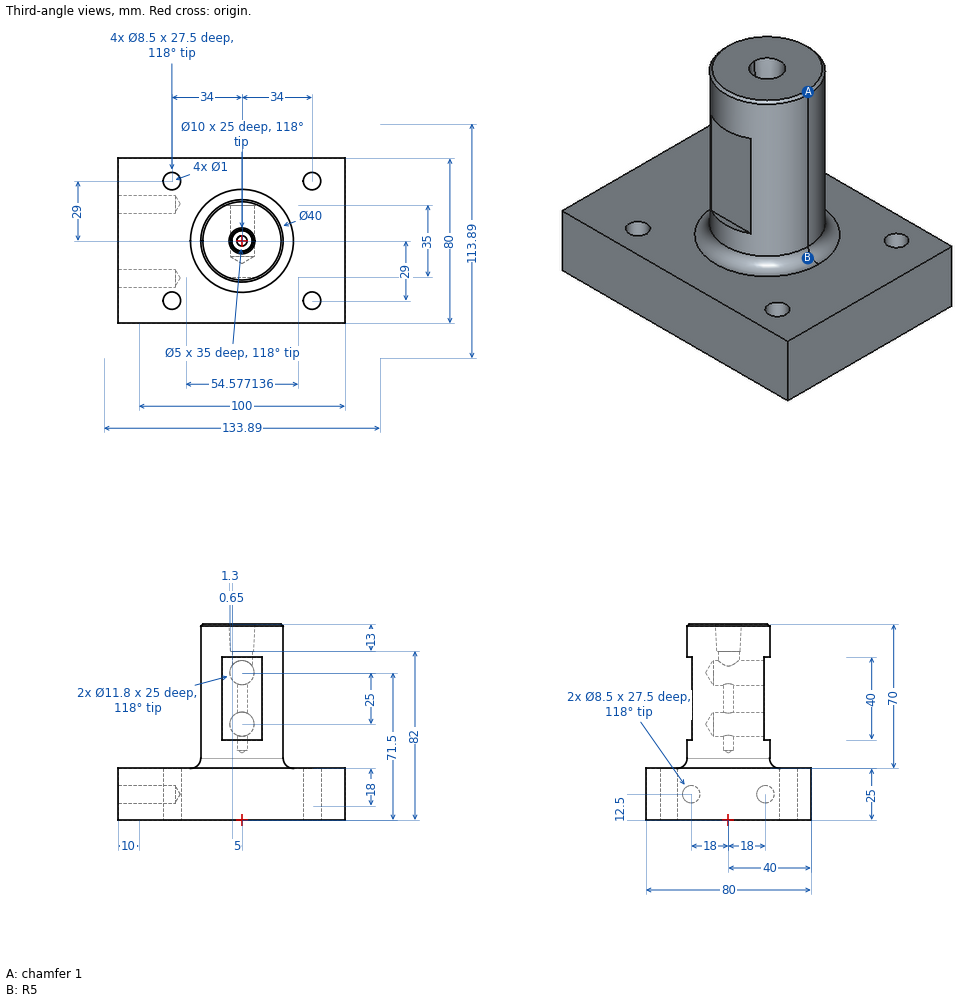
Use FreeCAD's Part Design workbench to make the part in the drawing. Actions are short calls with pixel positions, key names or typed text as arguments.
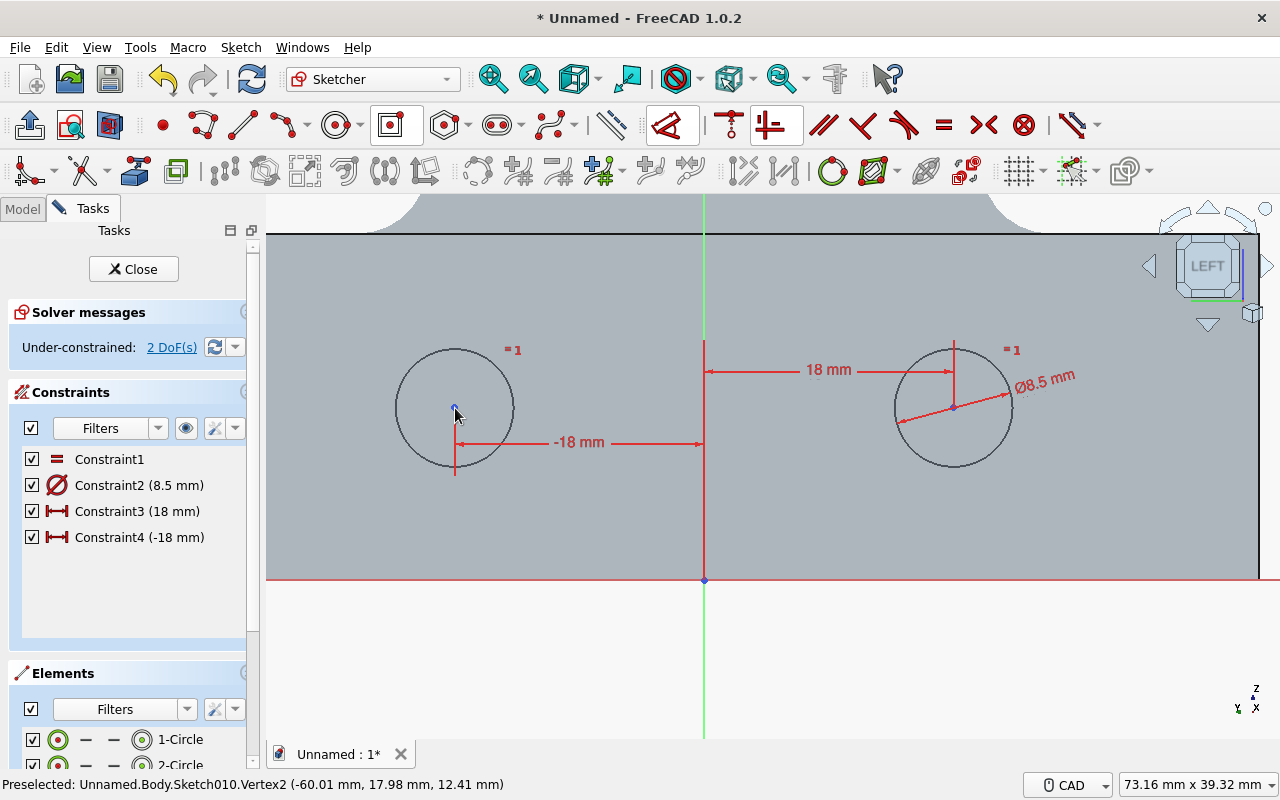
click(954, 408)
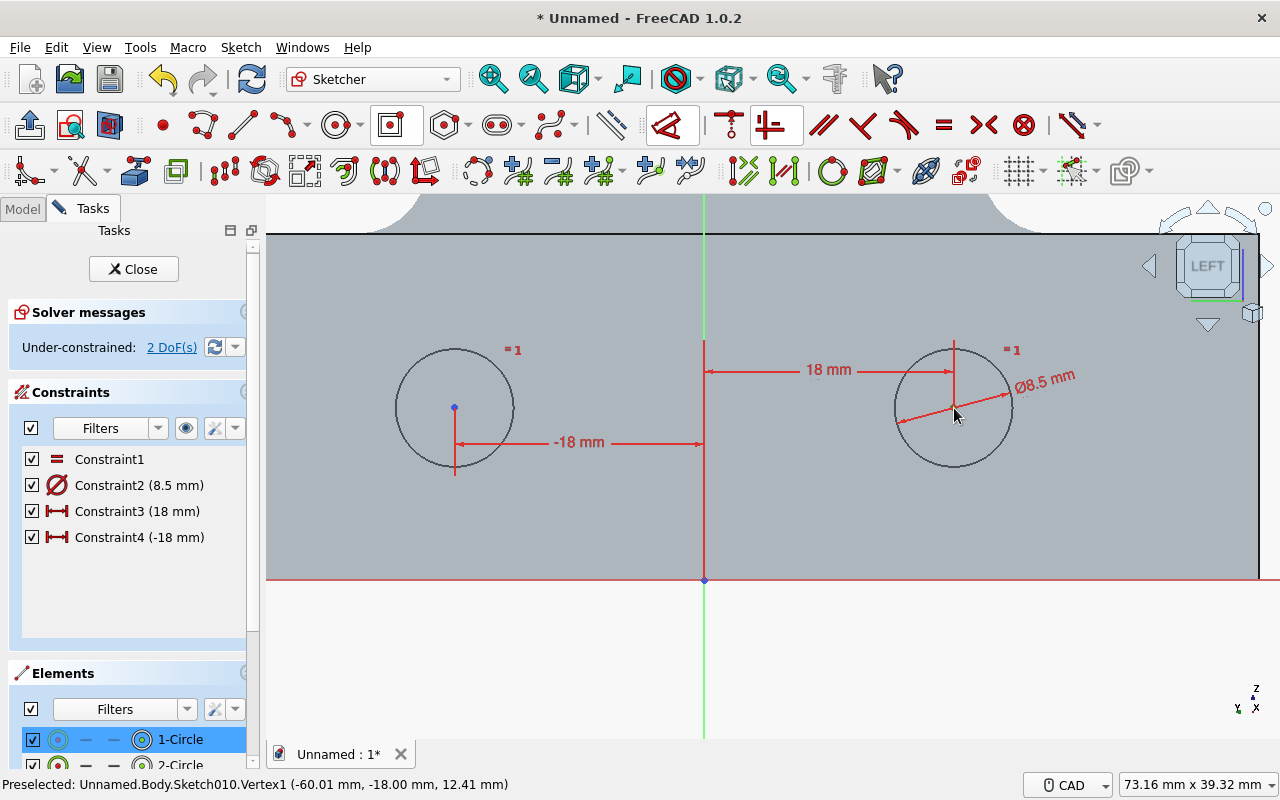
click(694, 126)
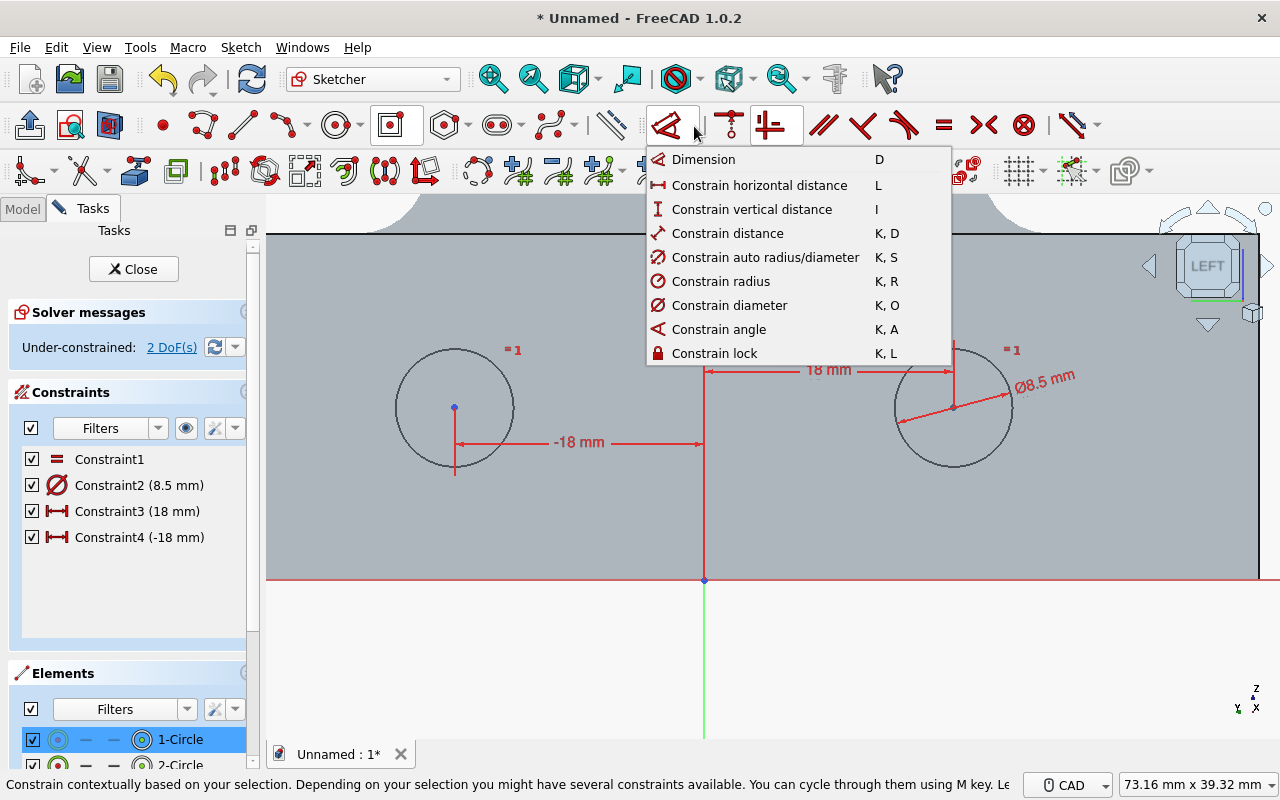
click(799, 209)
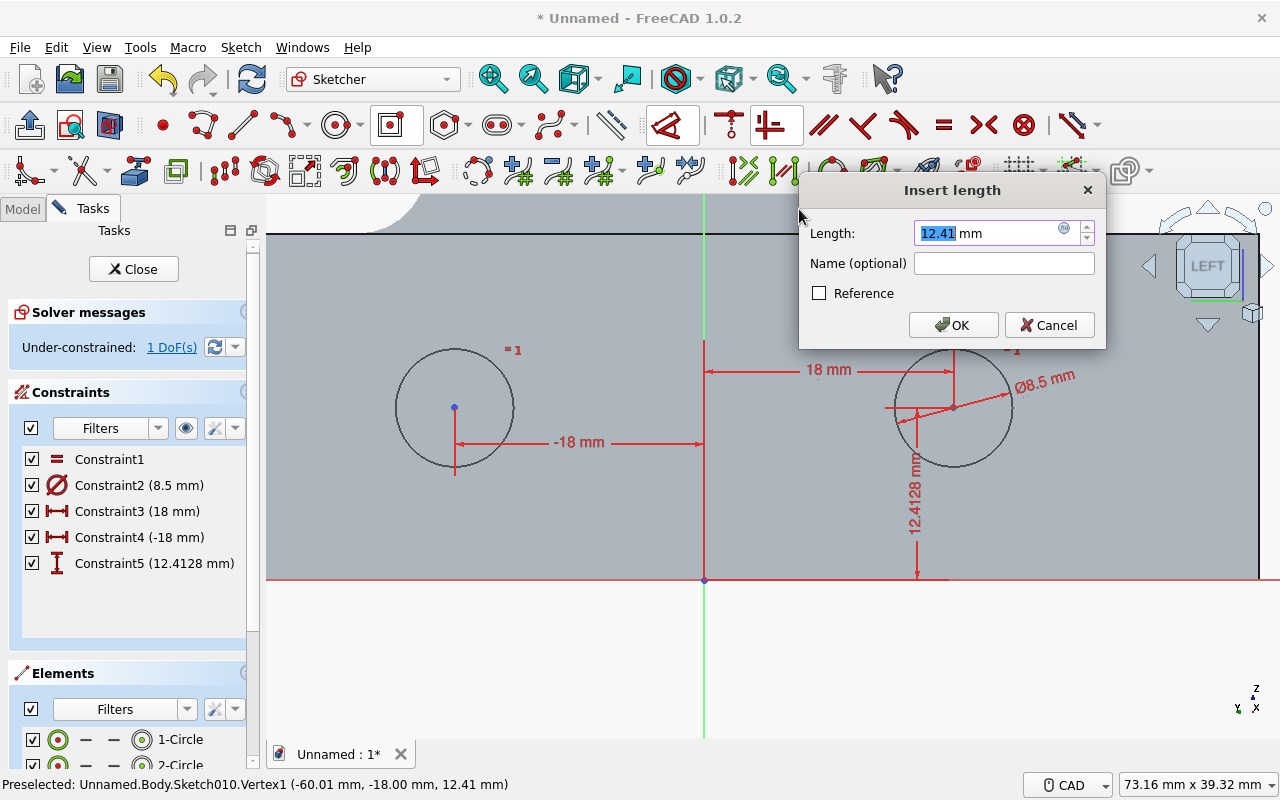
text(12.5)
key(Return)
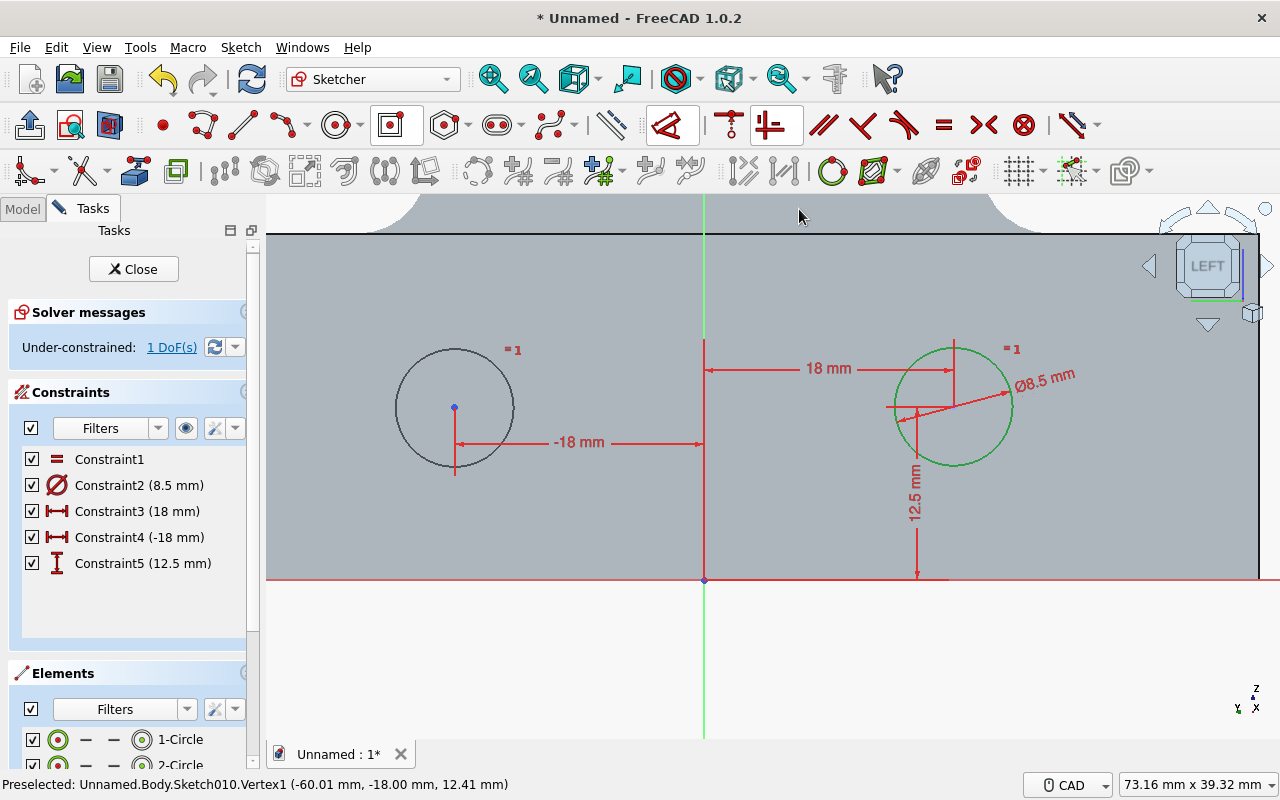
click(455, 408)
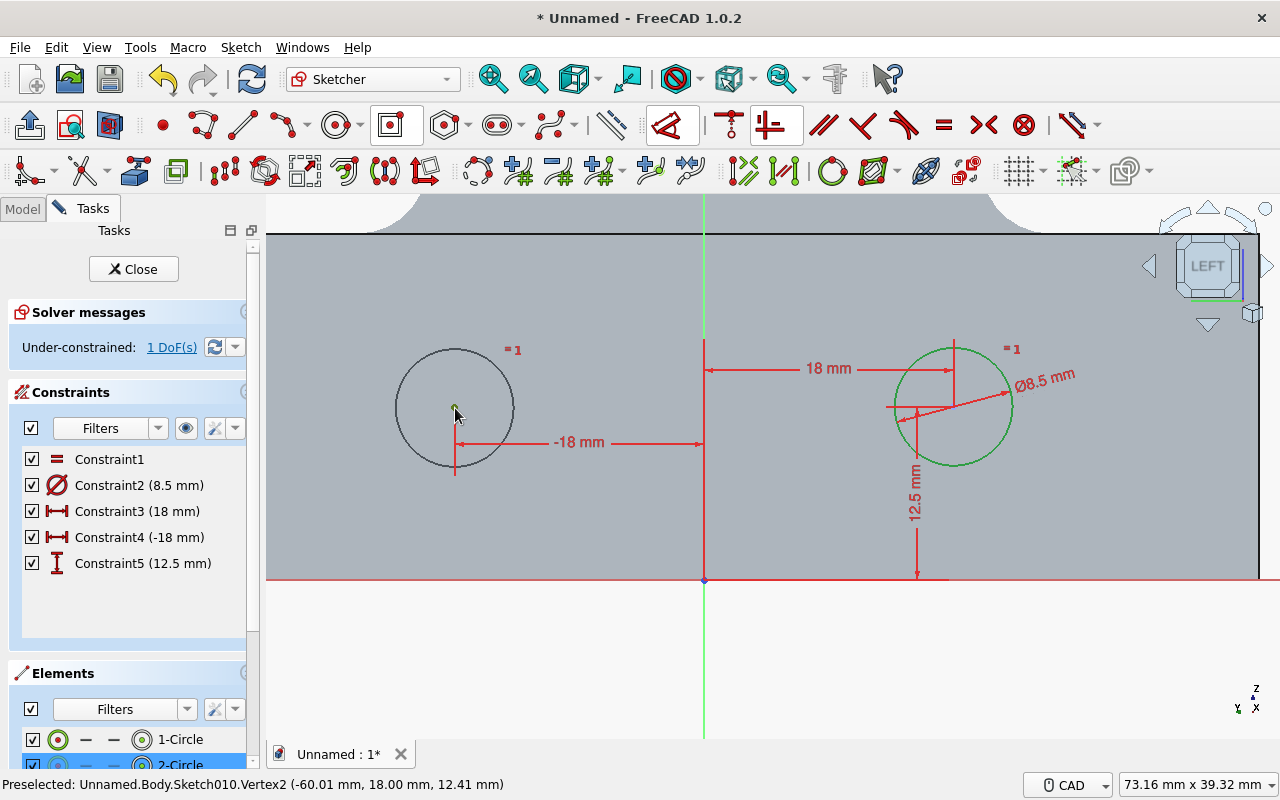
click(694, 126)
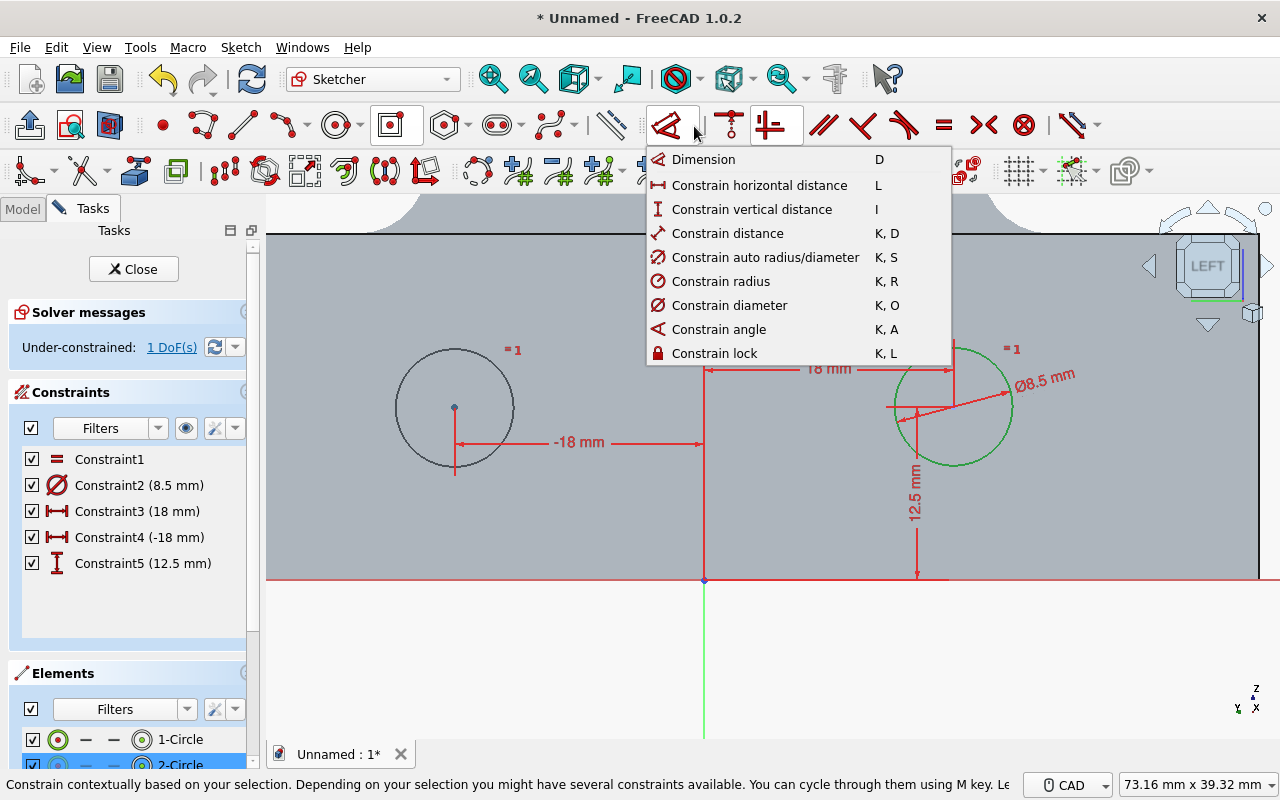
click(799, 209)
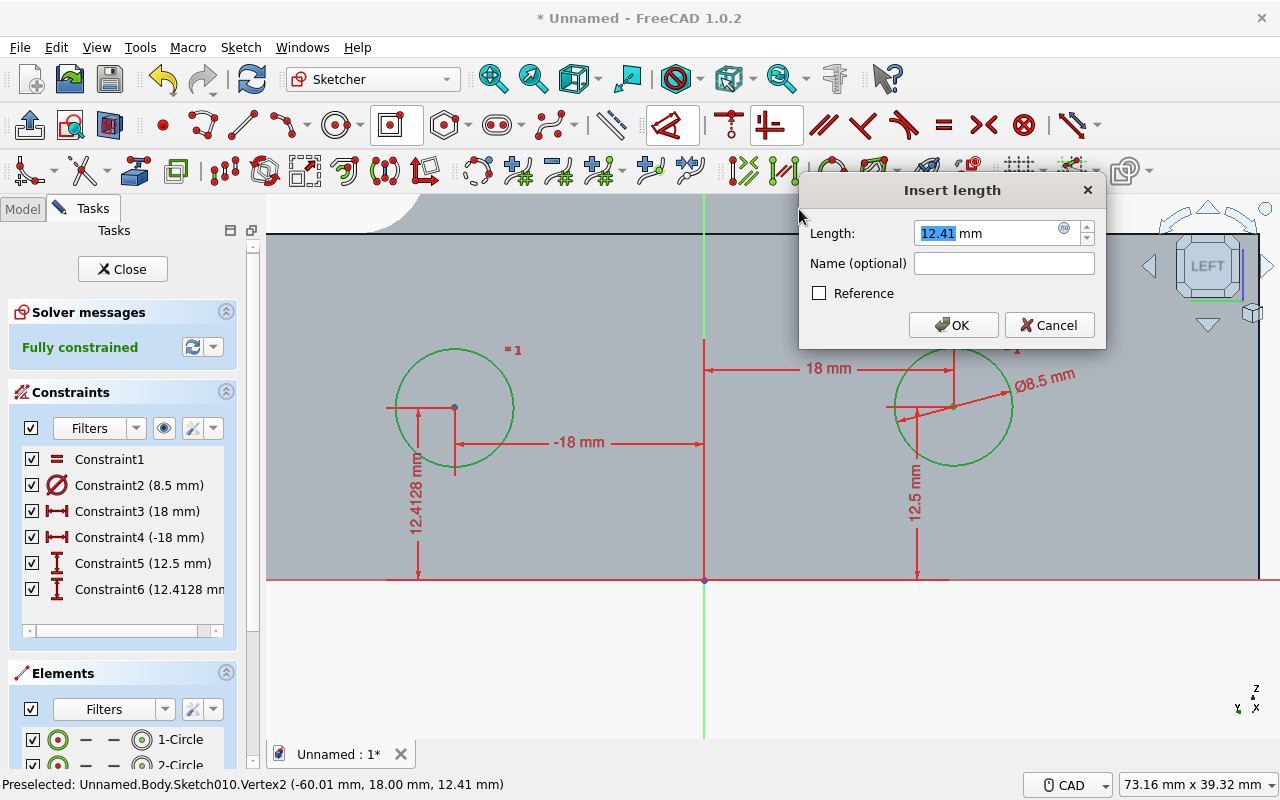
text(12.5)
key(Return)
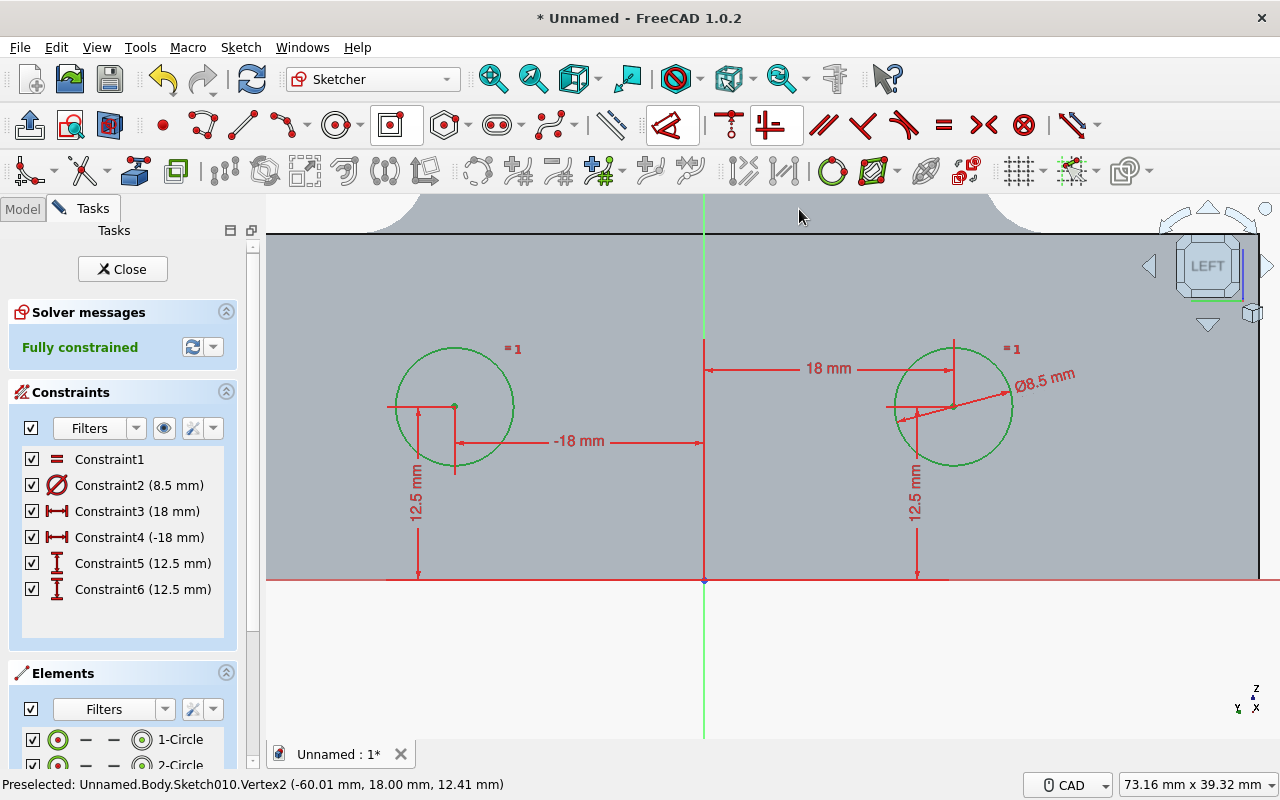
click(123, 269)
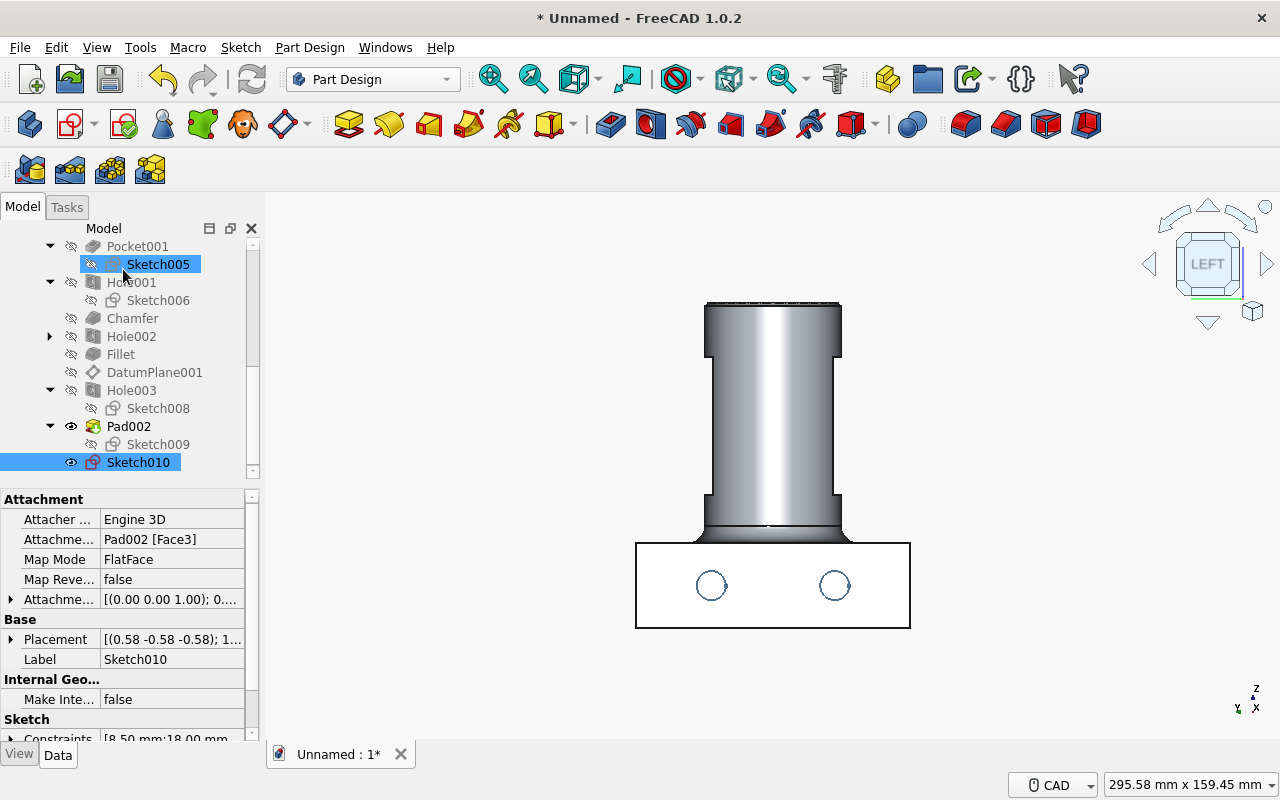
click(652, 124)